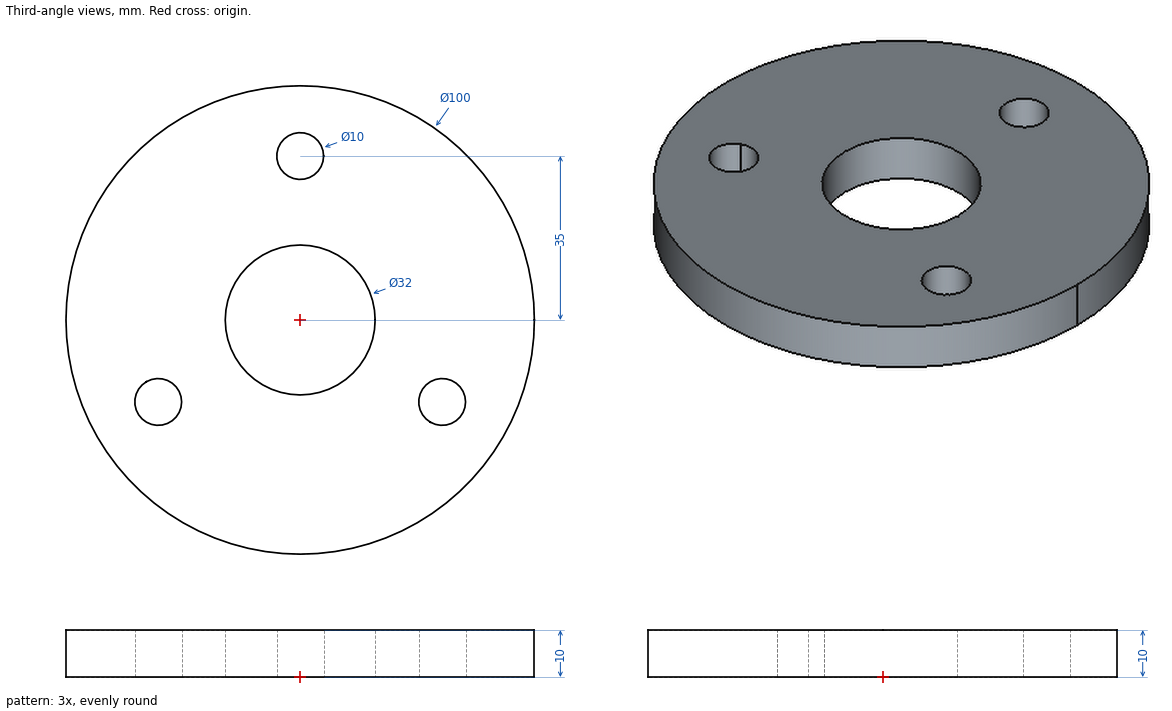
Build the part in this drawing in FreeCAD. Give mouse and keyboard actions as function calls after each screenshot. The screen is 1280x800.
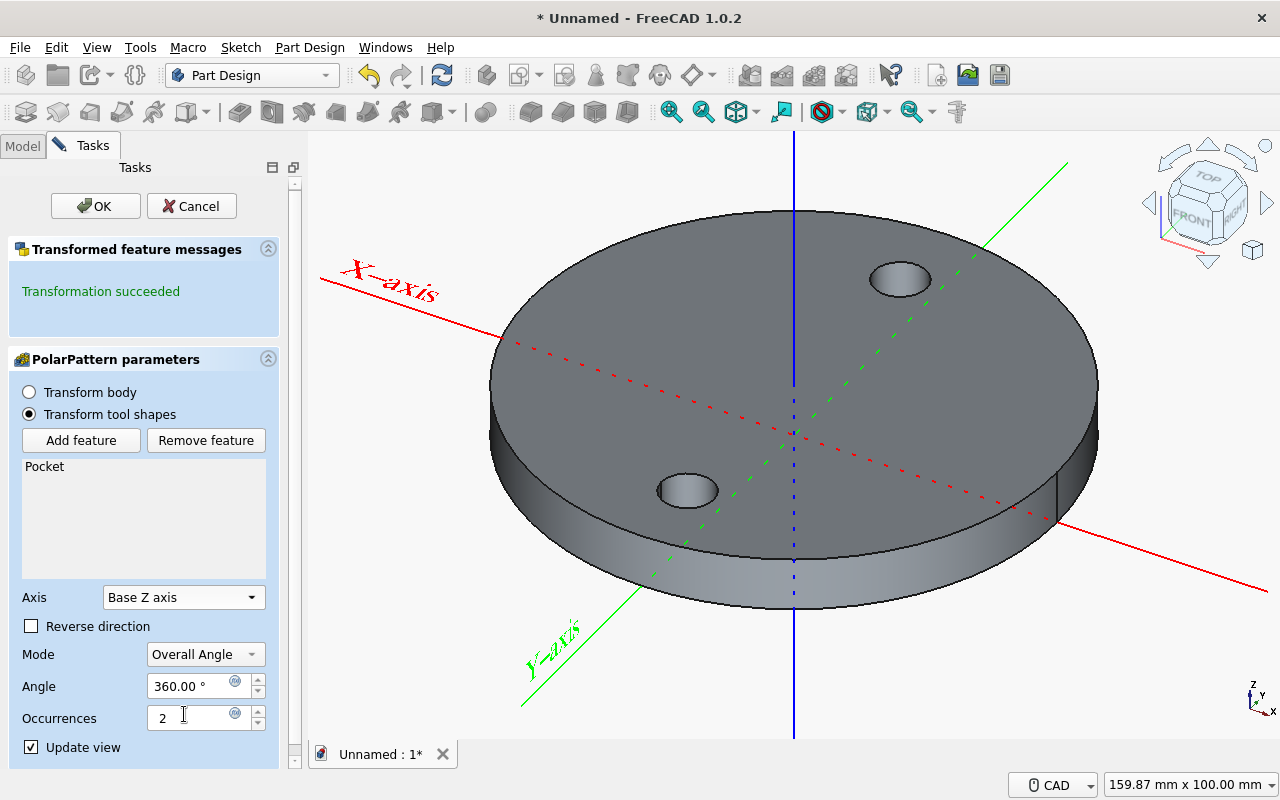
triple_click(198, 718)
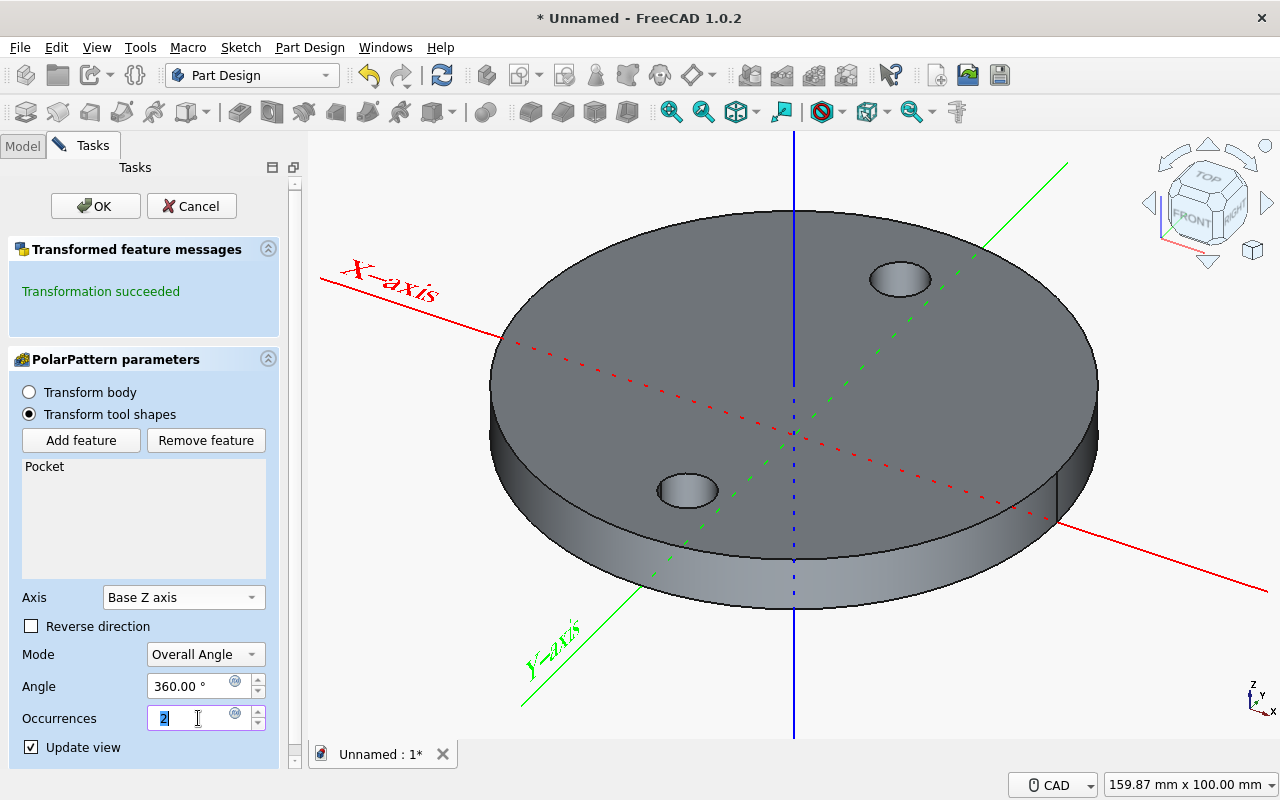
text(3)
key(Tab)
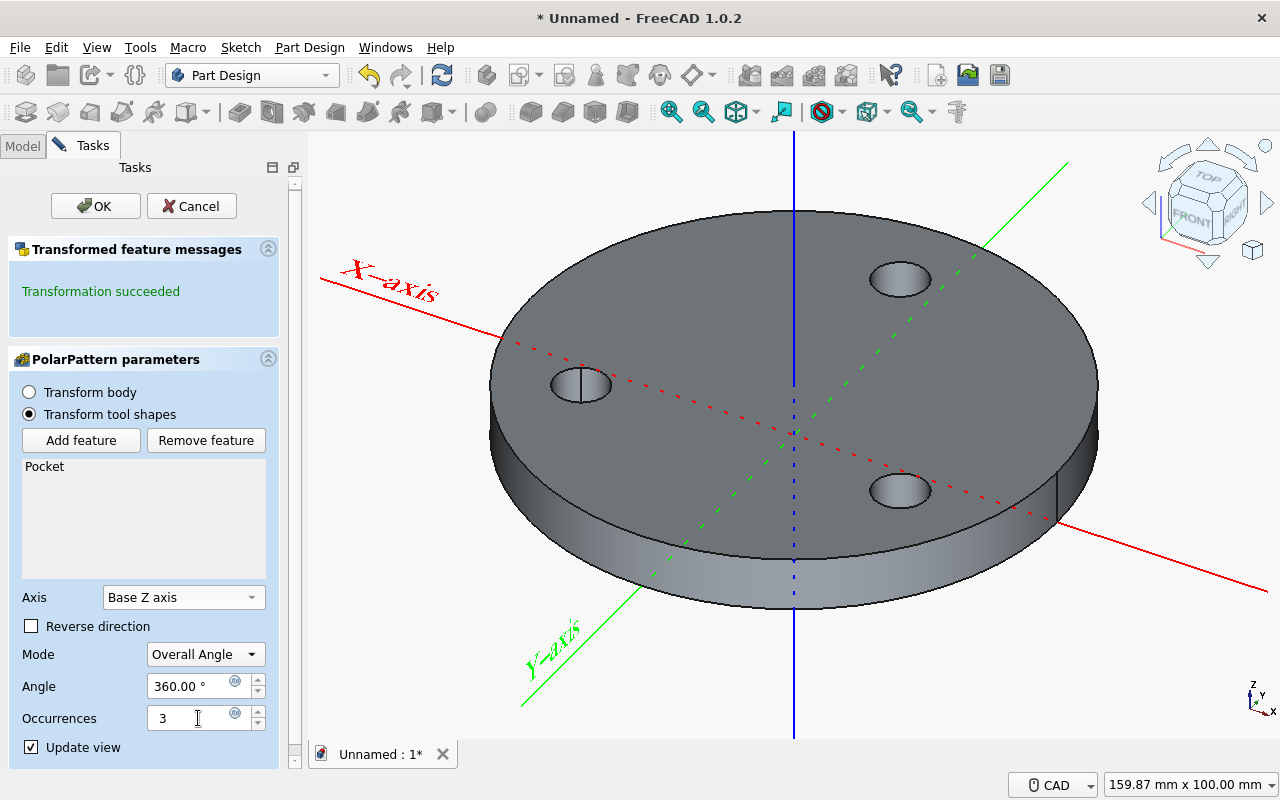
click(96, 206)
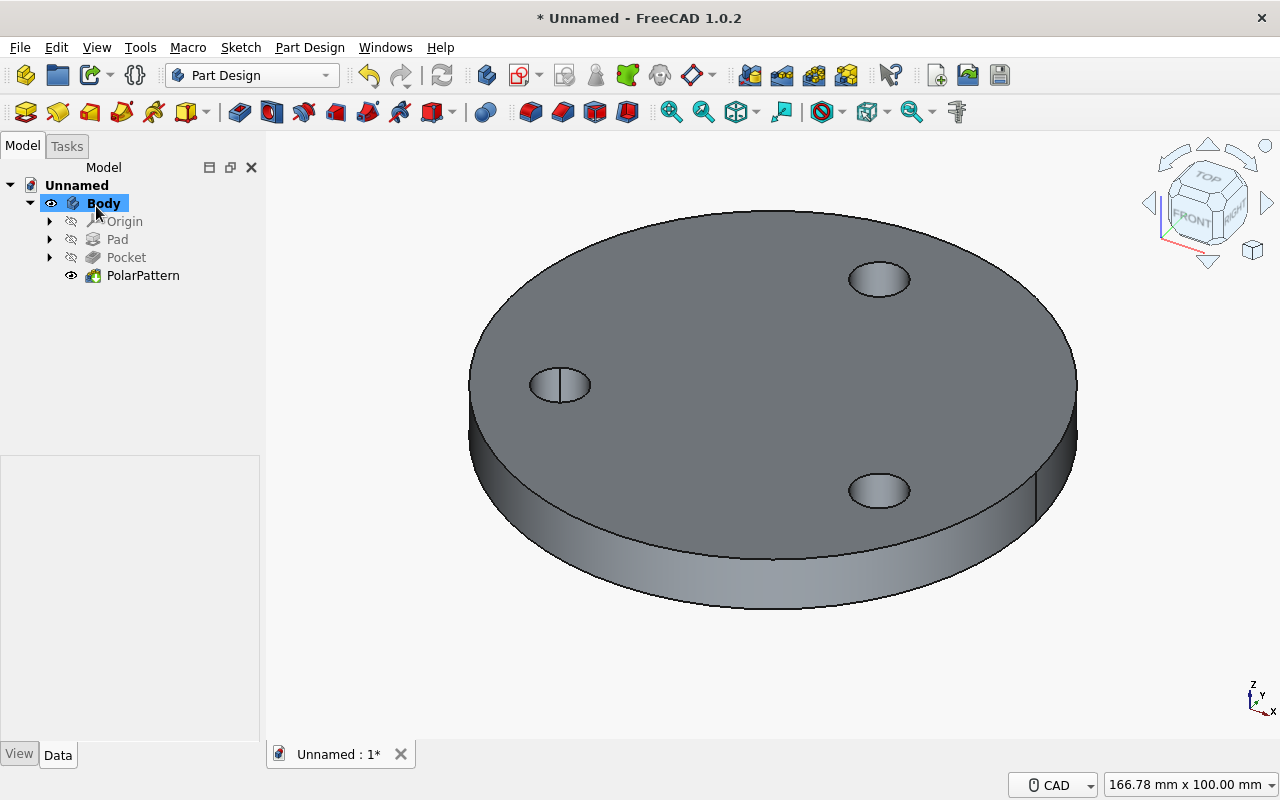
click(773, 384)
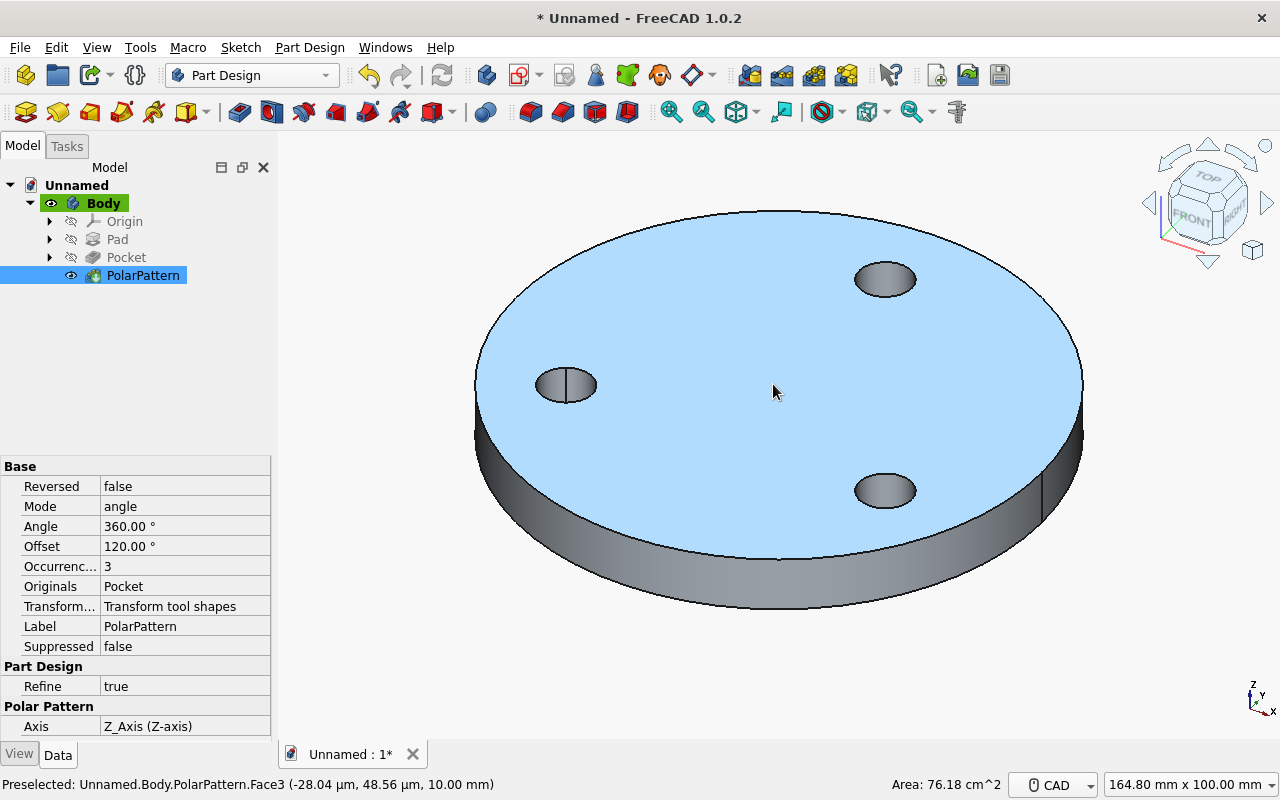
click(520, 76)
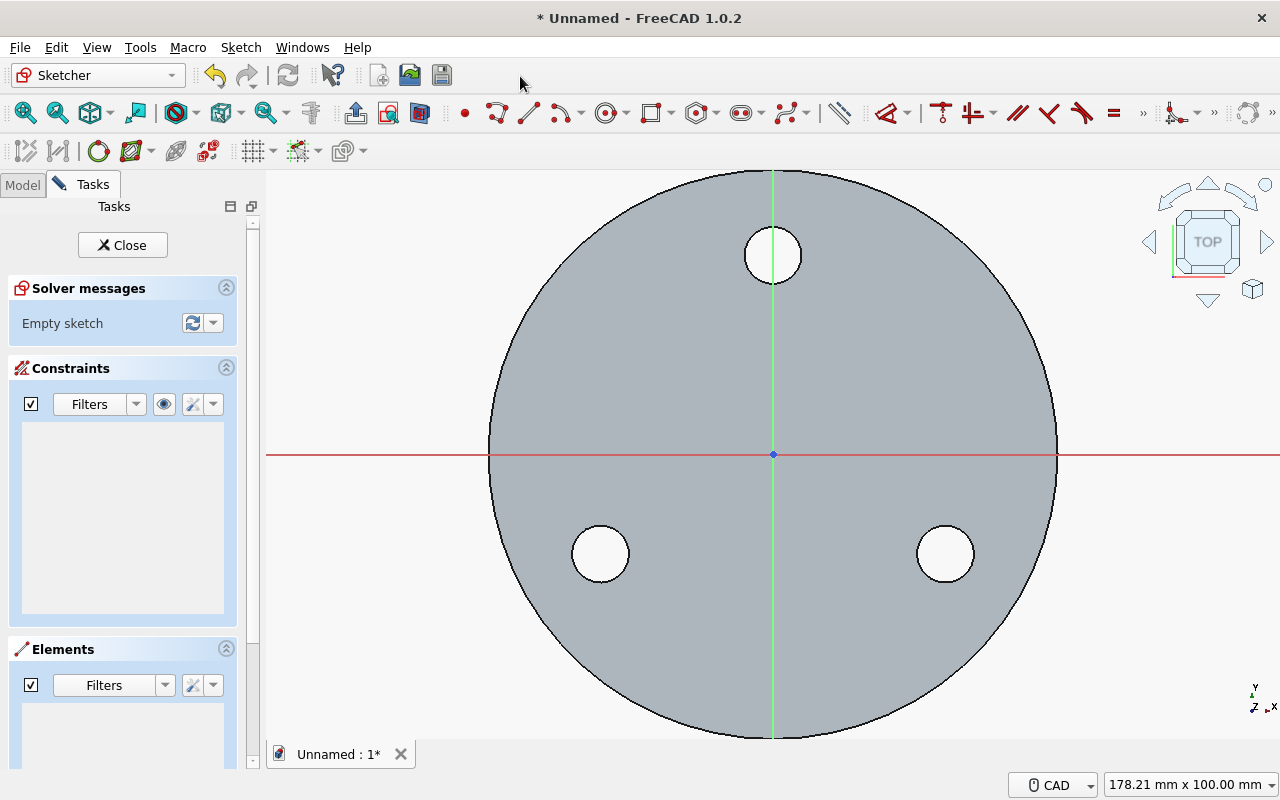
scroll(856, 454, up, 3)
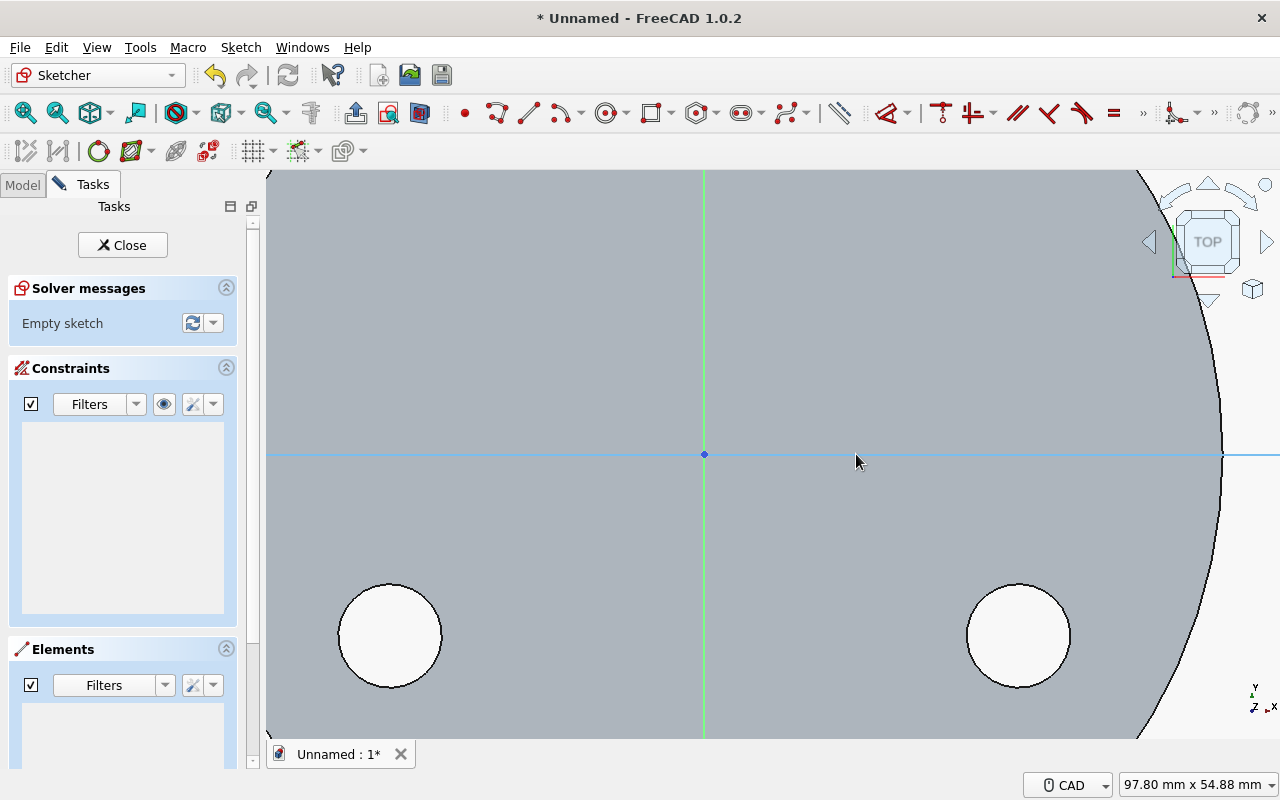
click(606, 114)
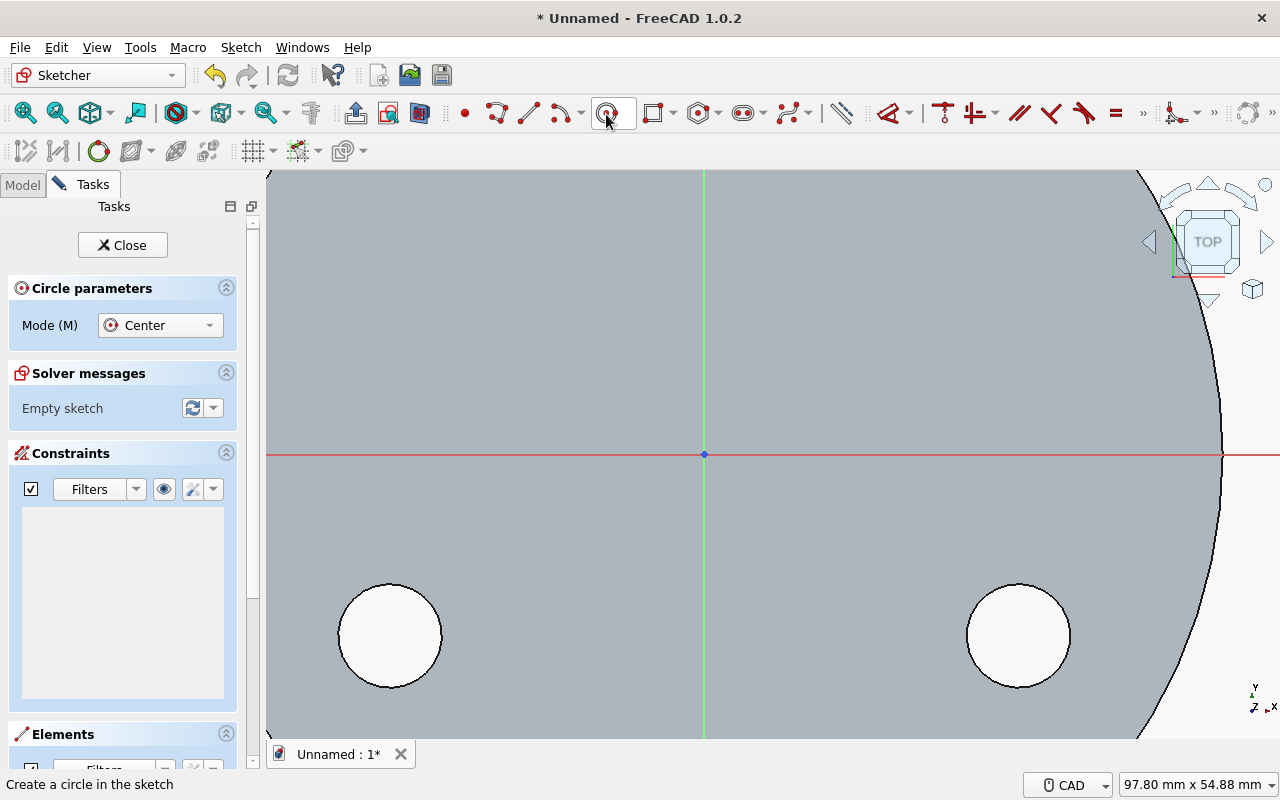
click(704, 454)
move(822, 337)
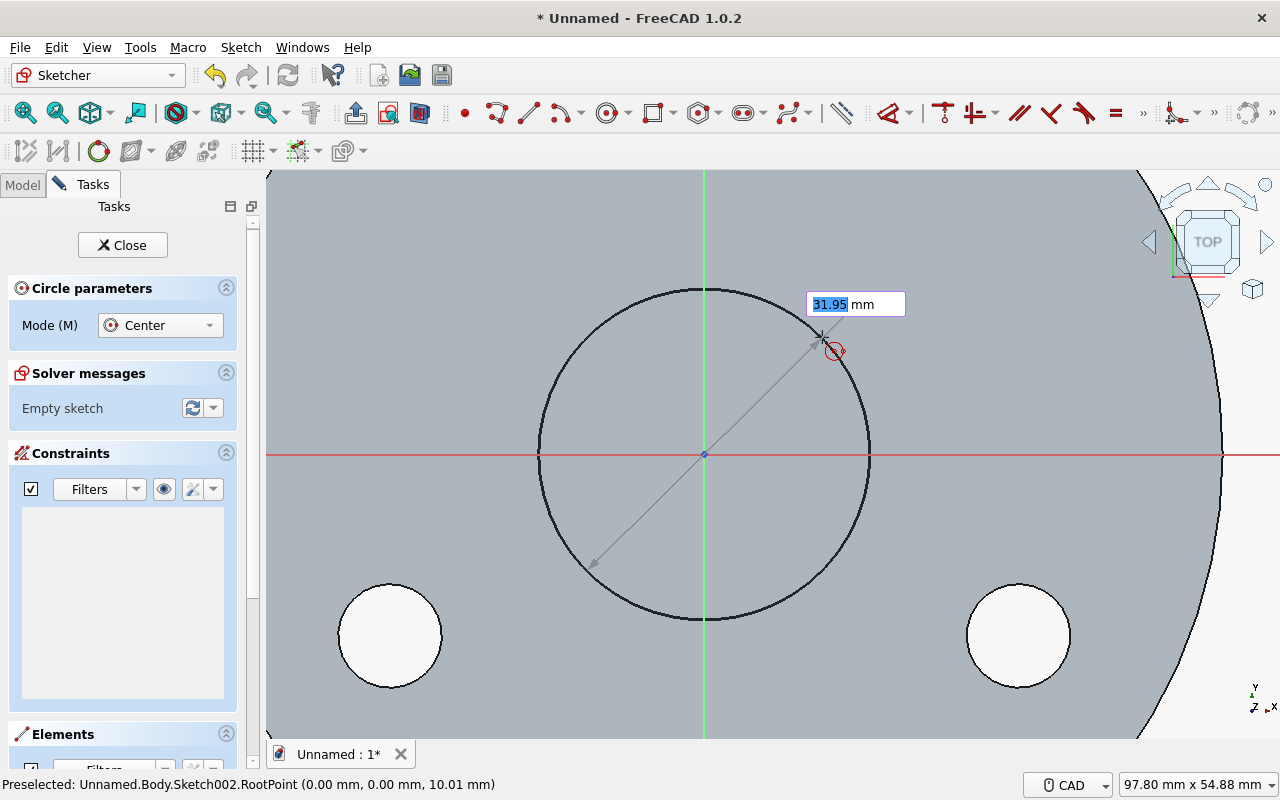
text(32)
key(Return)
key(Escape)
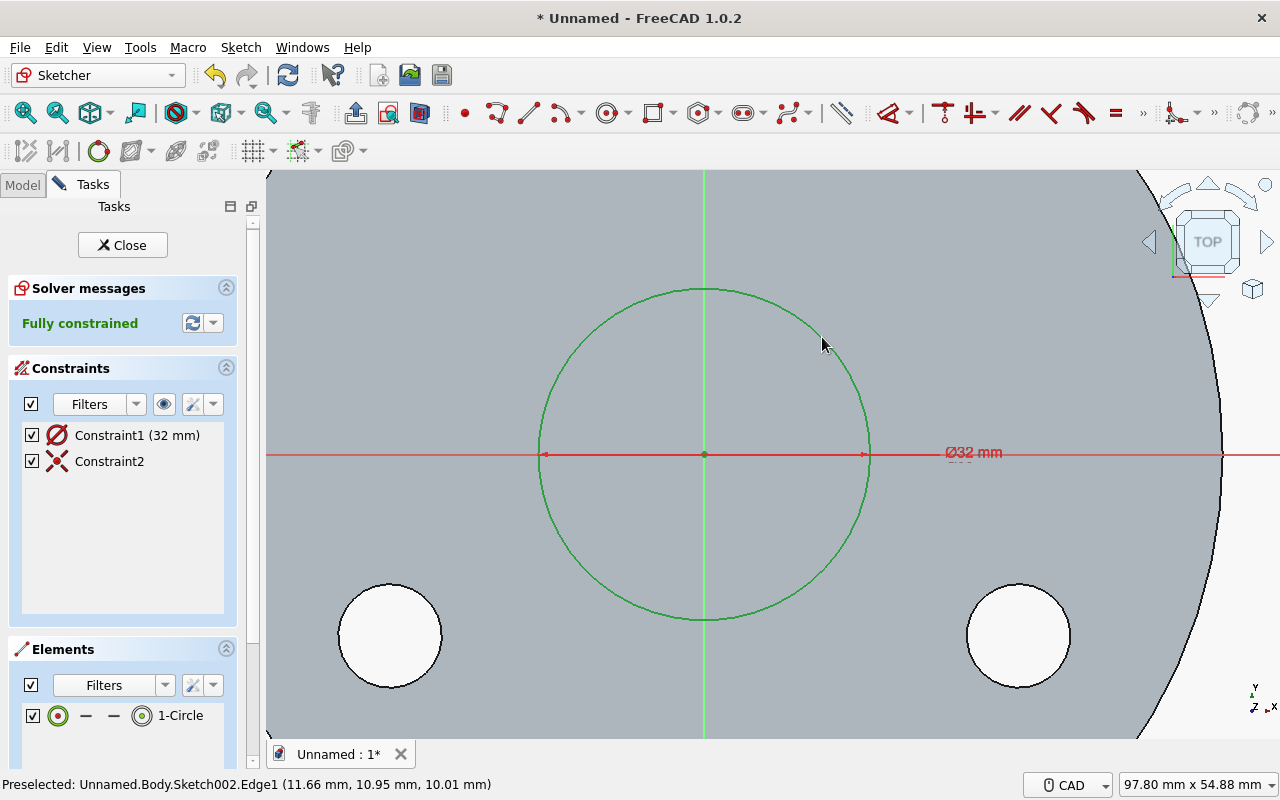
click(123, 245)